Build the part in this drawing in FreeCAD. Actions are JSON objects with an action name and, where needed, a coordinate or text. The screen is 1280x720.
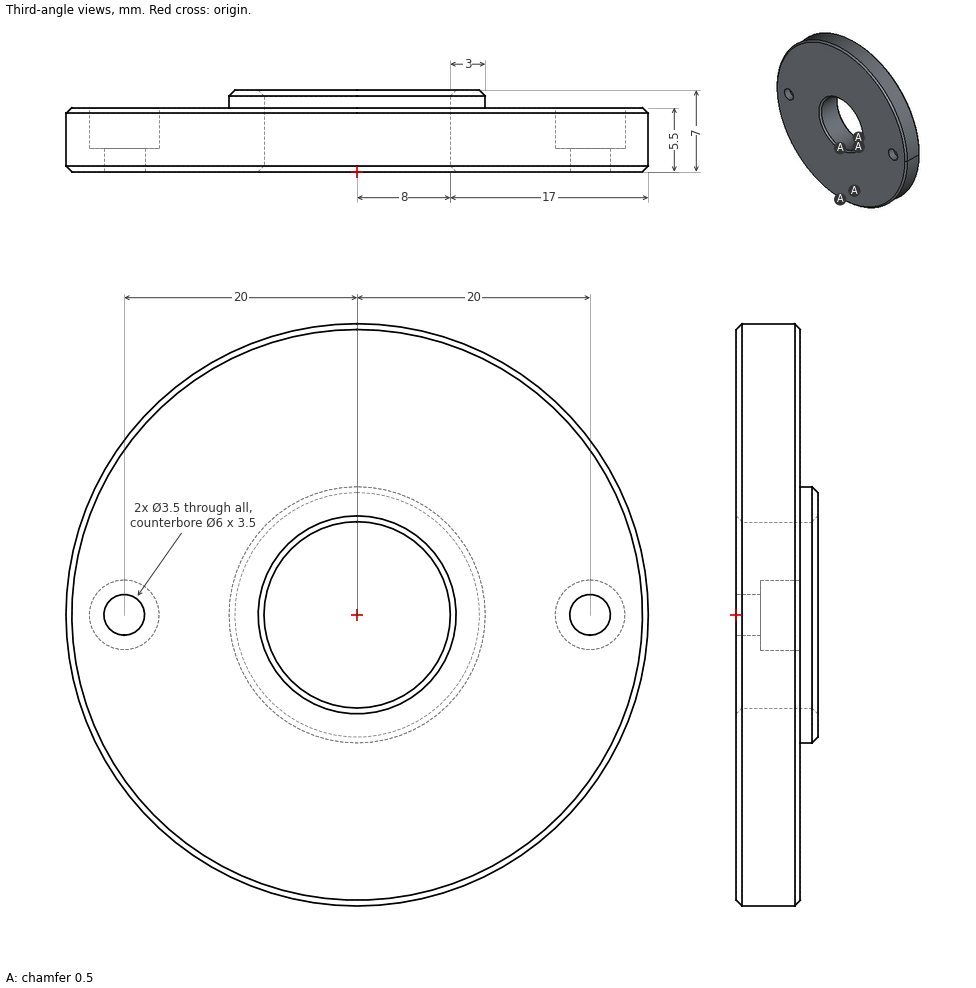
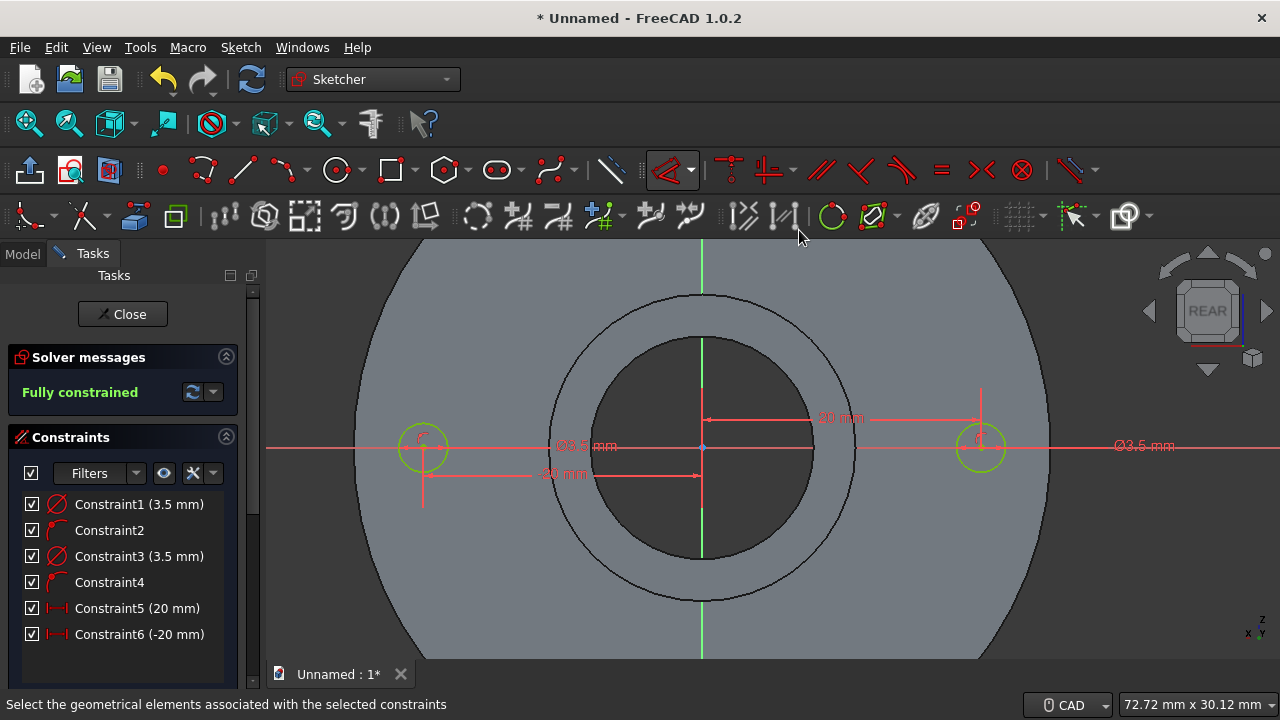
{"action": "left_click", "coordinate": [123, 314]}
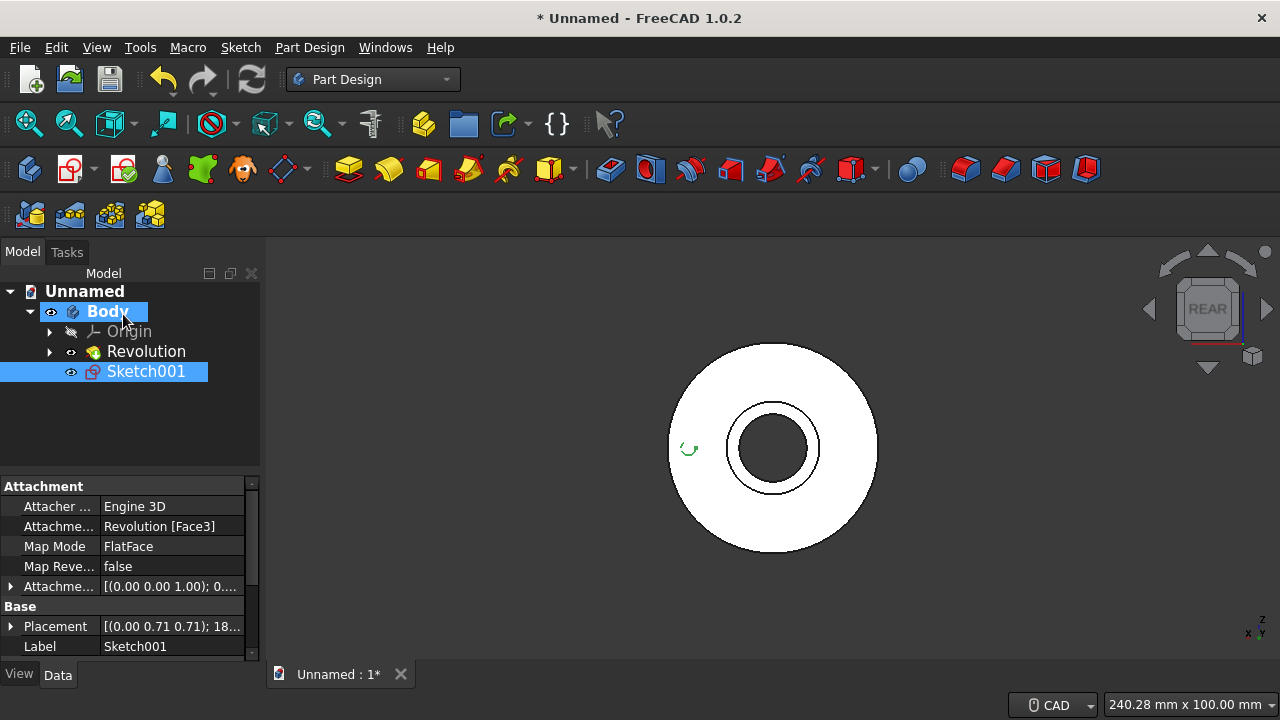
{"action": "left_click", "coordinate": [652, 170]}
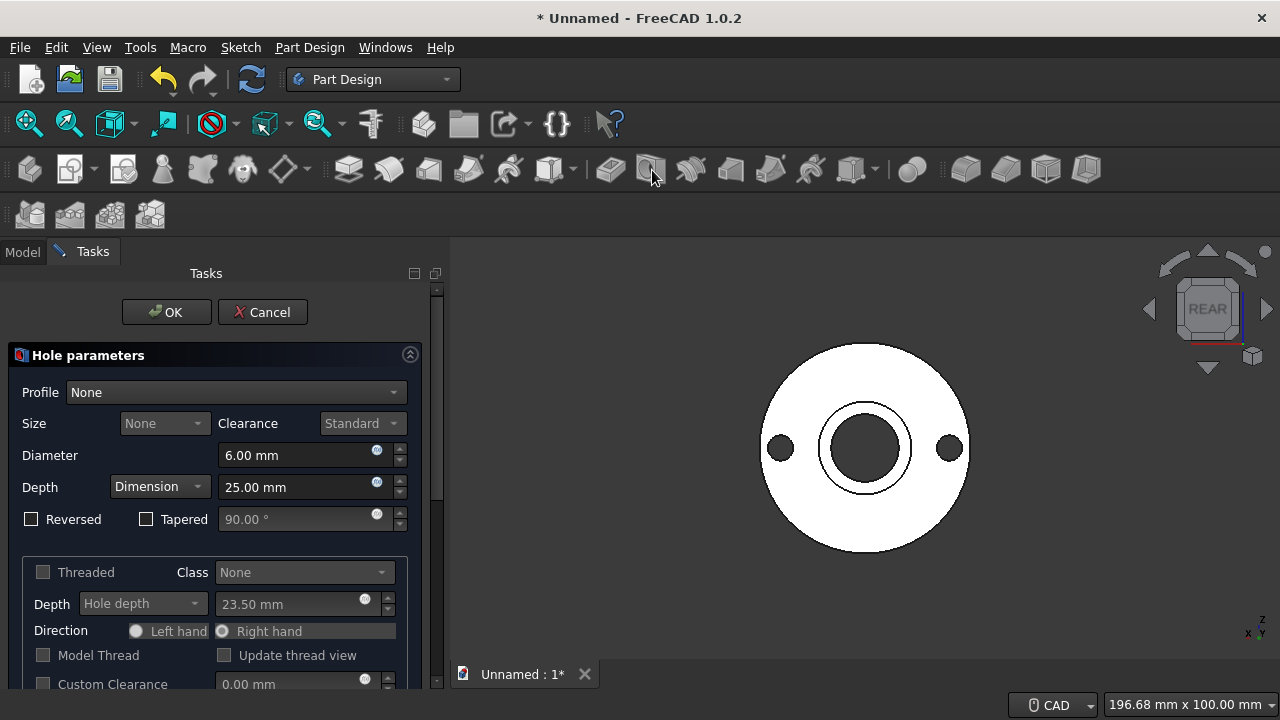
{"action": "triple_click", "coordinate": [305, 455]}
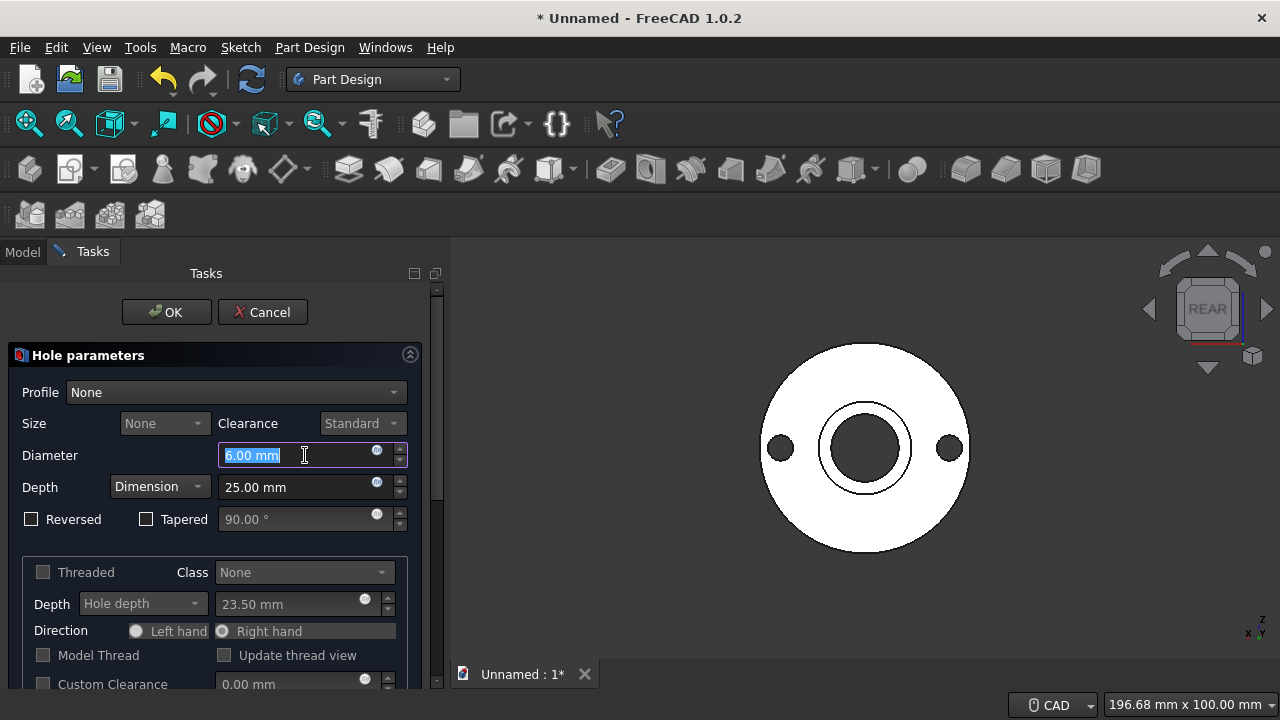
{"action": "type", "text": "3.5"}
{"action": "key", "text": "Tab"}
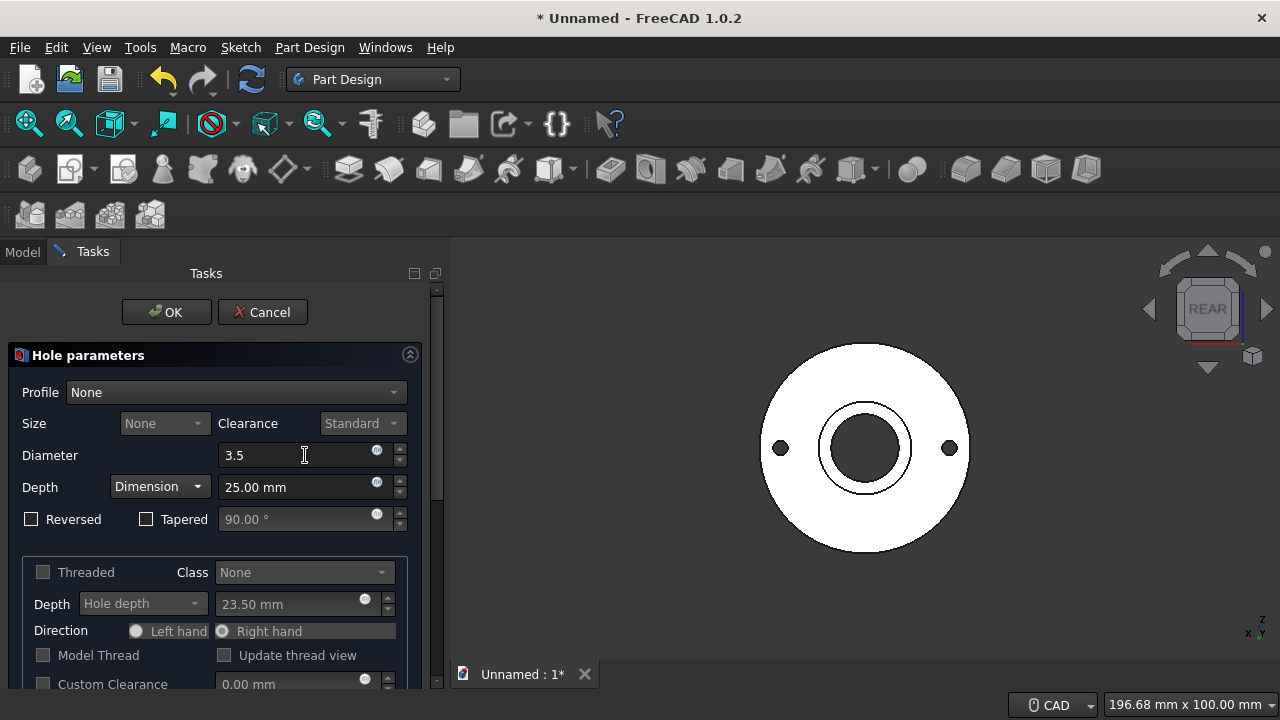
{"action": "left_click", "coordinate": [161, 486]}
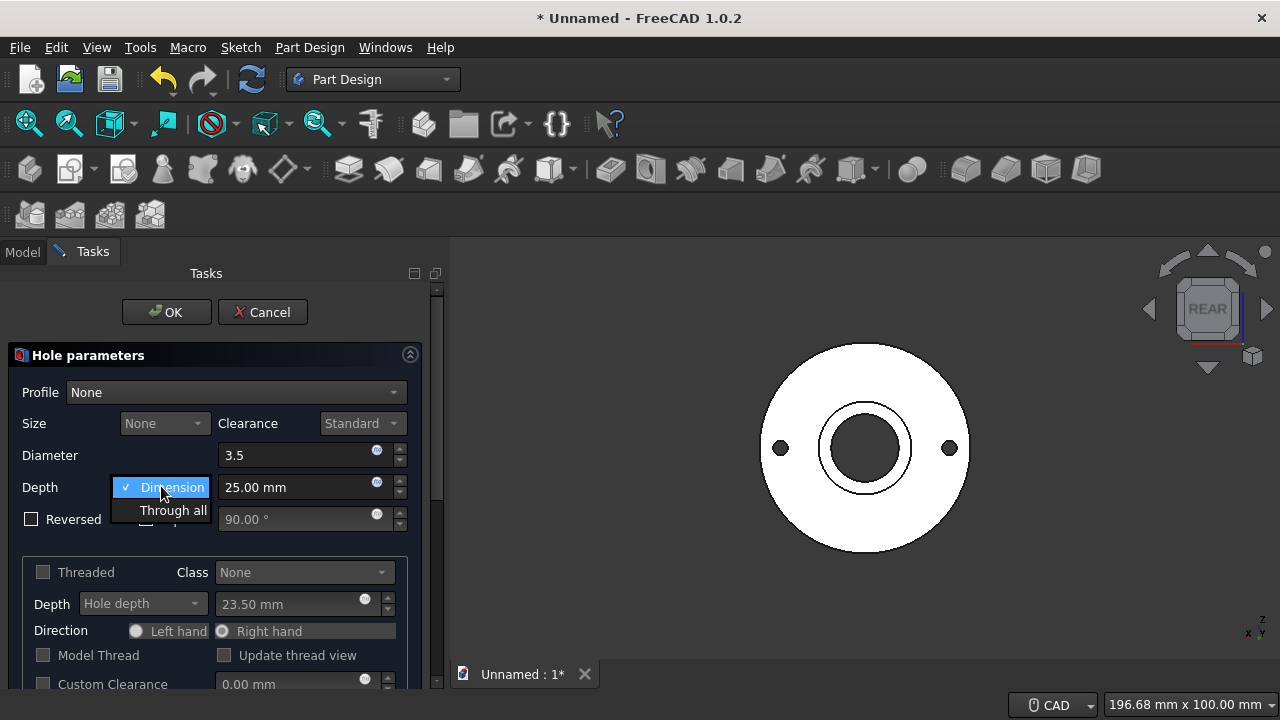
{"action": "left_click", "coordinate": [160, 510]}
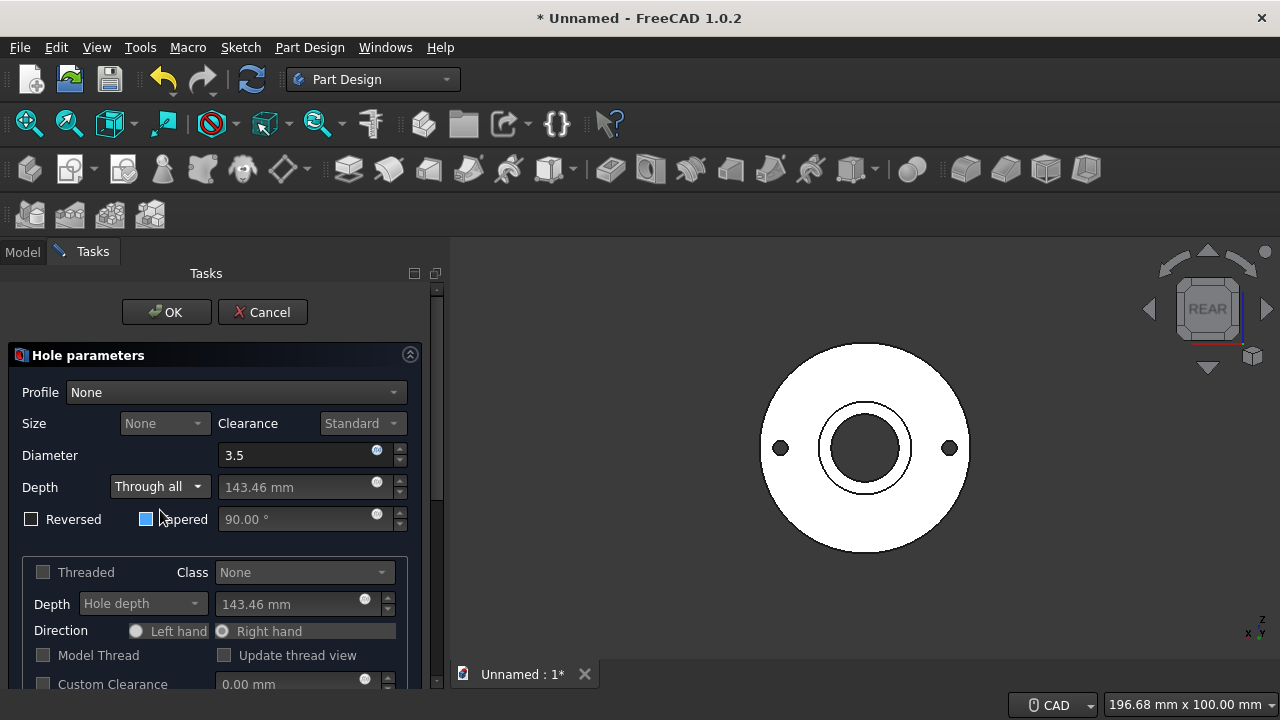
{"action": "scroll", "coordinate": [437, 486], "scroll_direction": "down", "scroll_amount": 3}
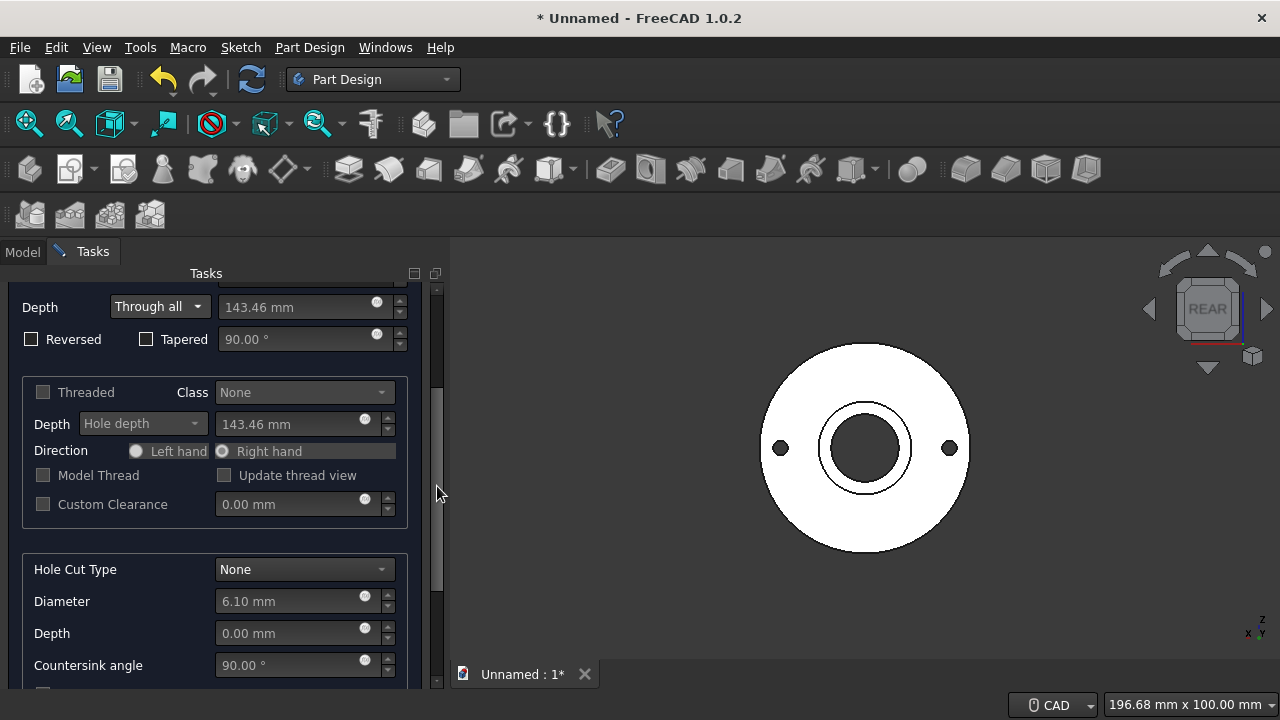
{"action": "left_click", "coordinate": [306, 570]}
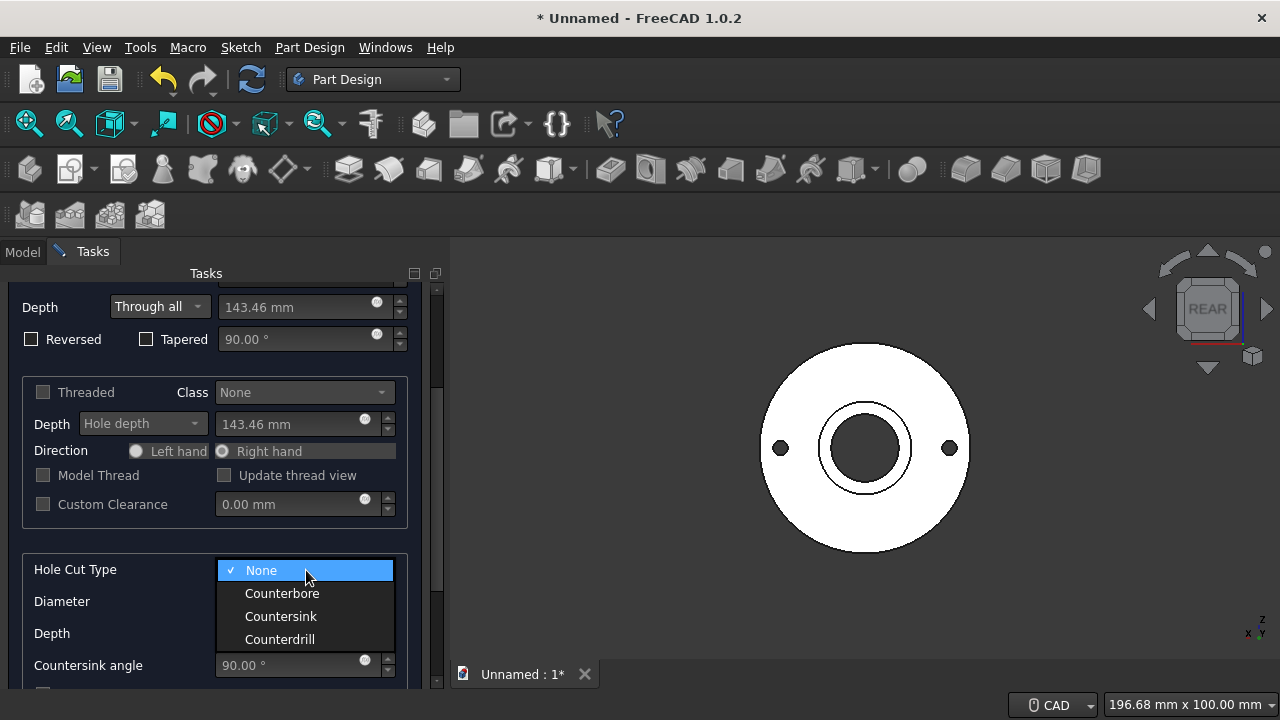
{"action": "left_click", "coordinate": [304, 594]}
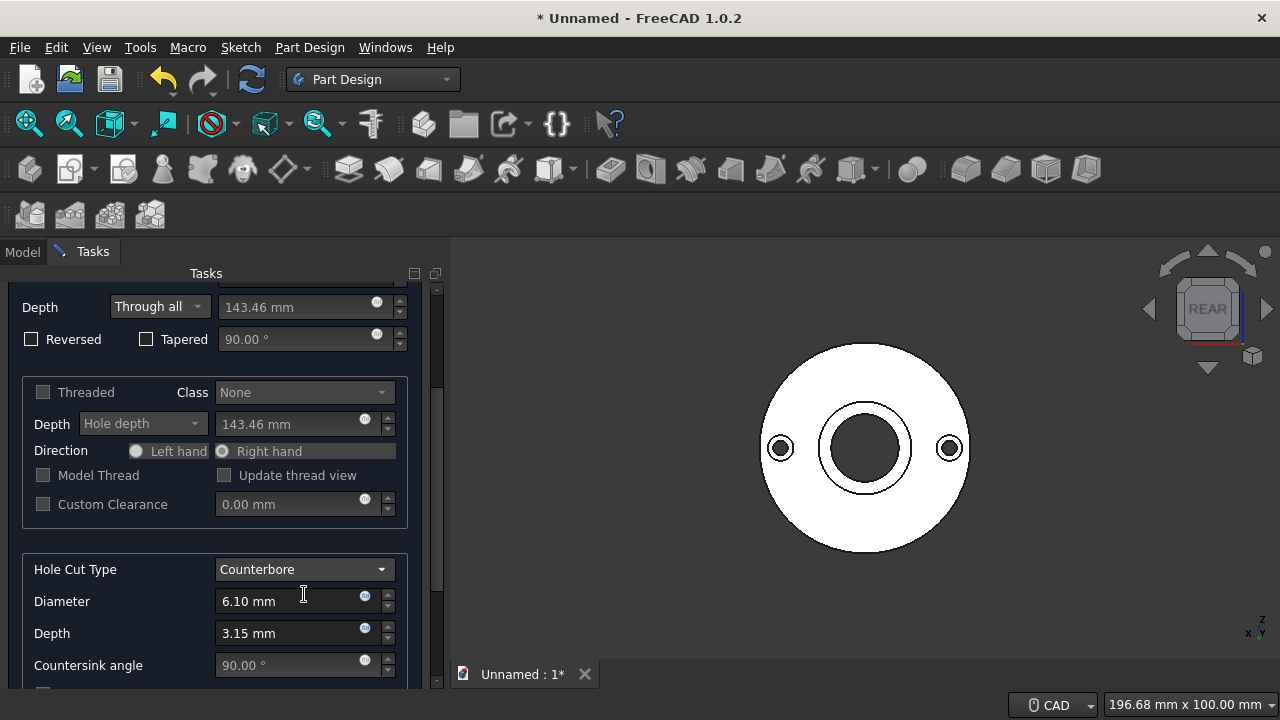
{"action": "triple_click", "coordinate": [298, 601]}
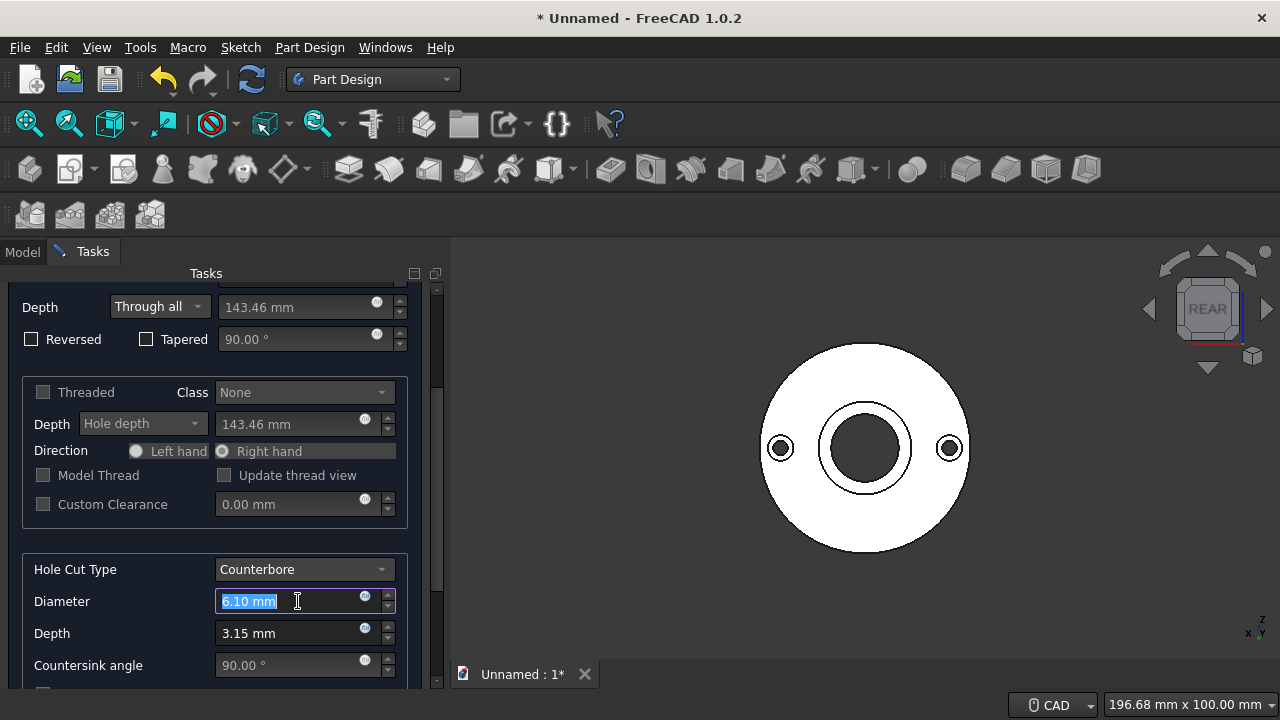
{"action": "type", "text": "6"}
{"action": "key", "text": "Tab"}